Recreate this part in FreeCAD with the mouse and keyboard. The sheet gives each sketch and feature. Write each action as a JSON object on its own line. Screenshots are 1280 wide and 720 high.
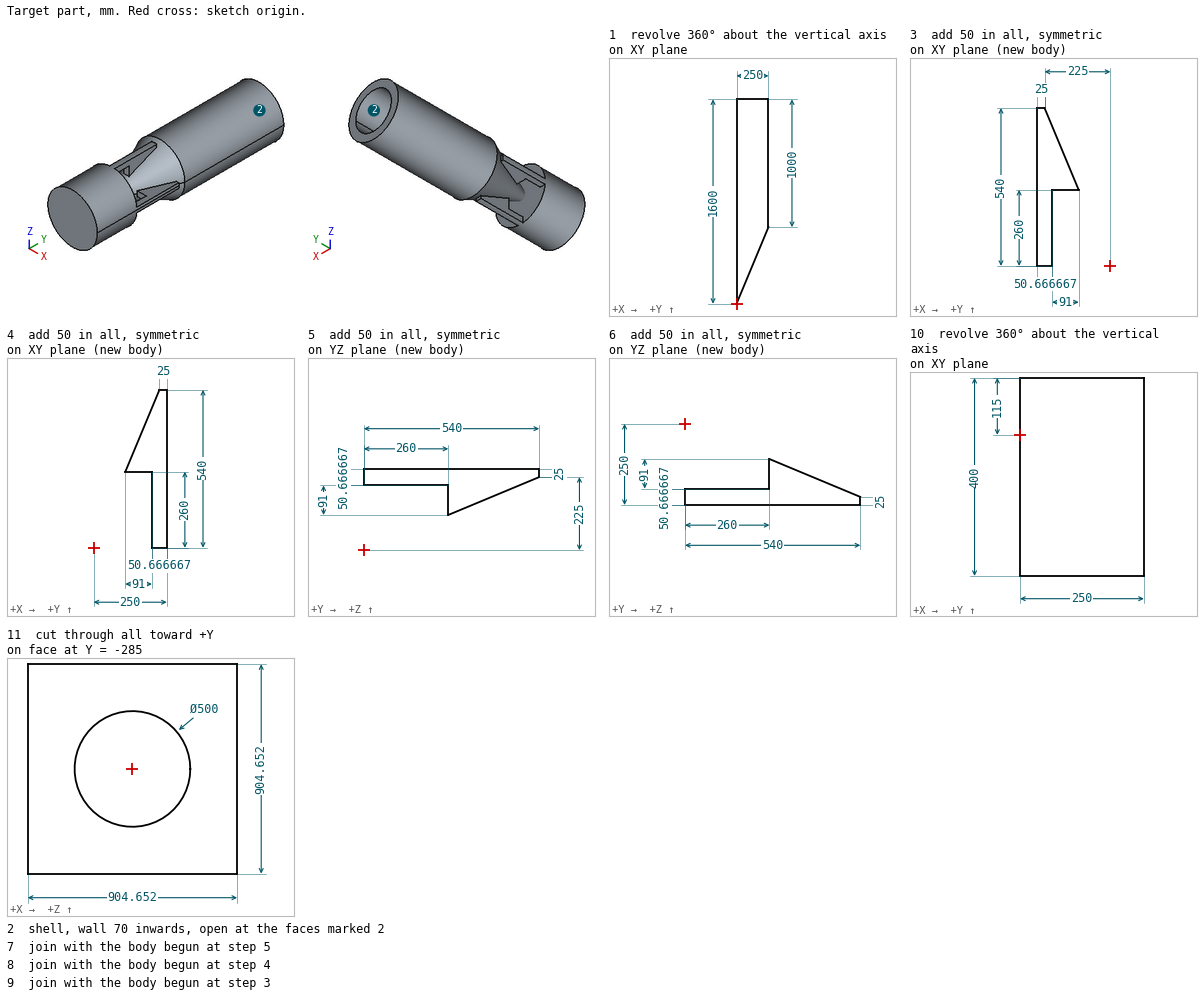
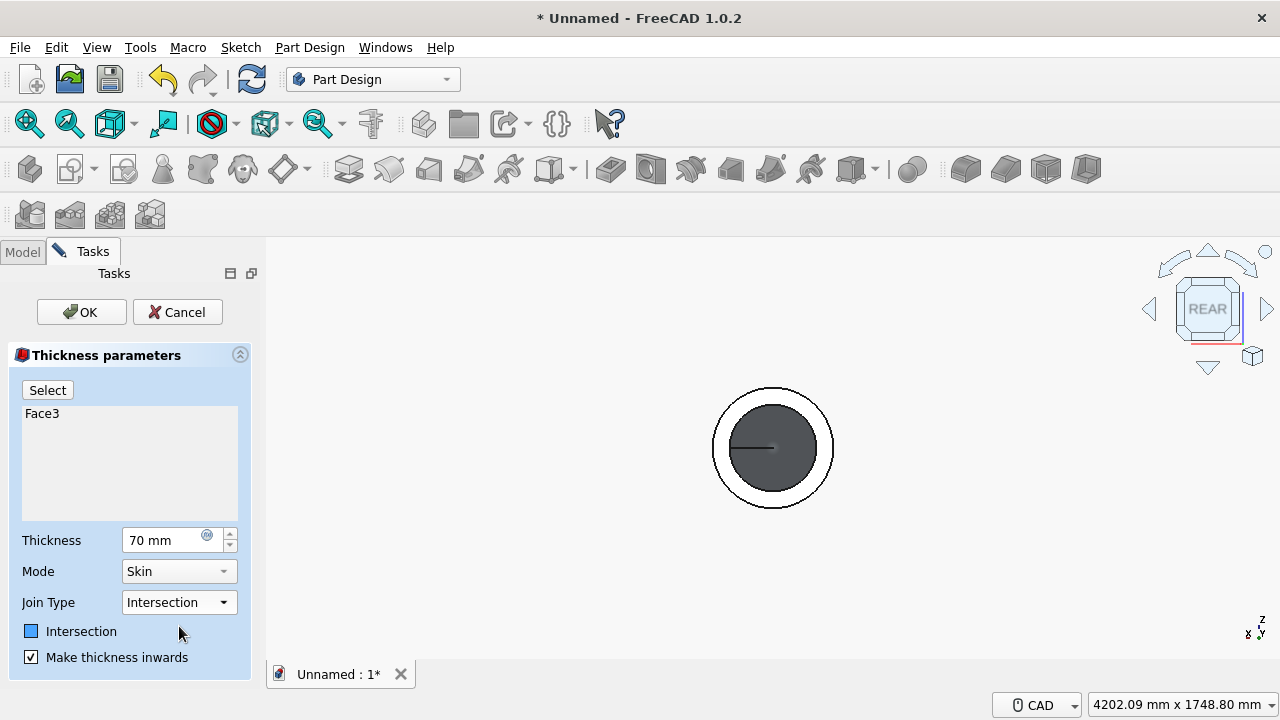
{"action": "left_click", "coordinate": [82, 312]}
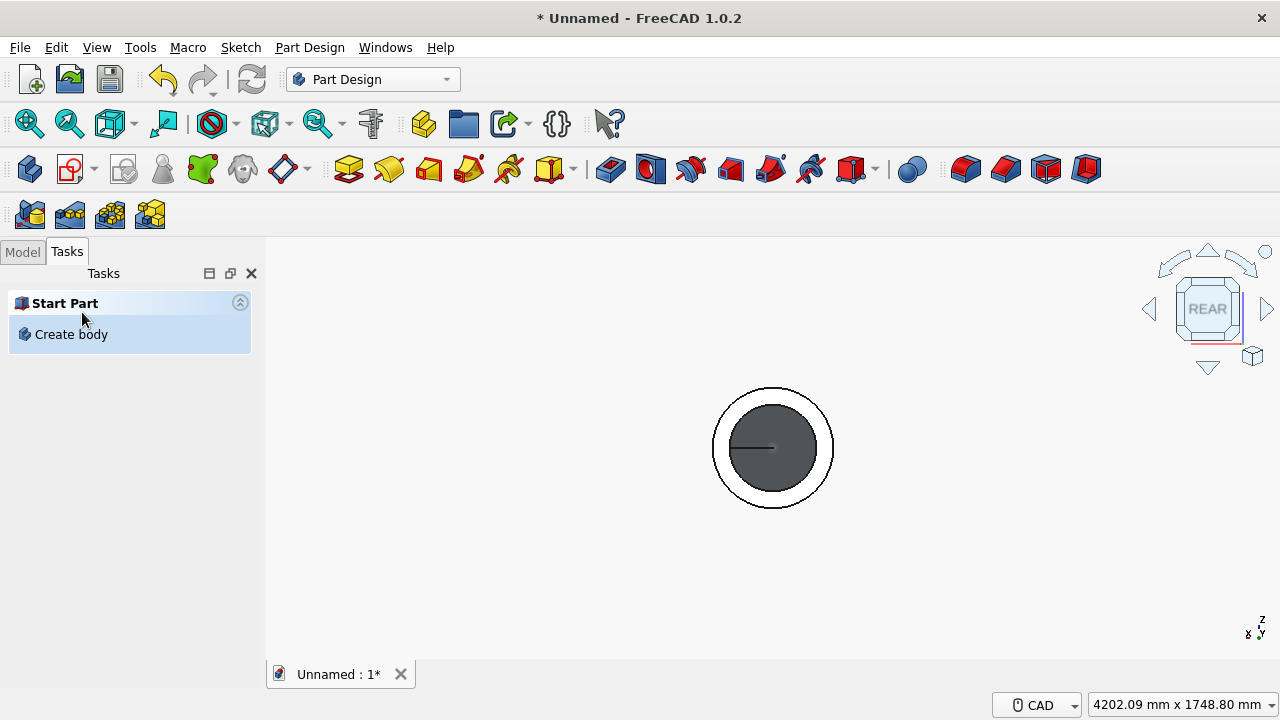
{"action": "left_click", "coordinate": [30, 124]}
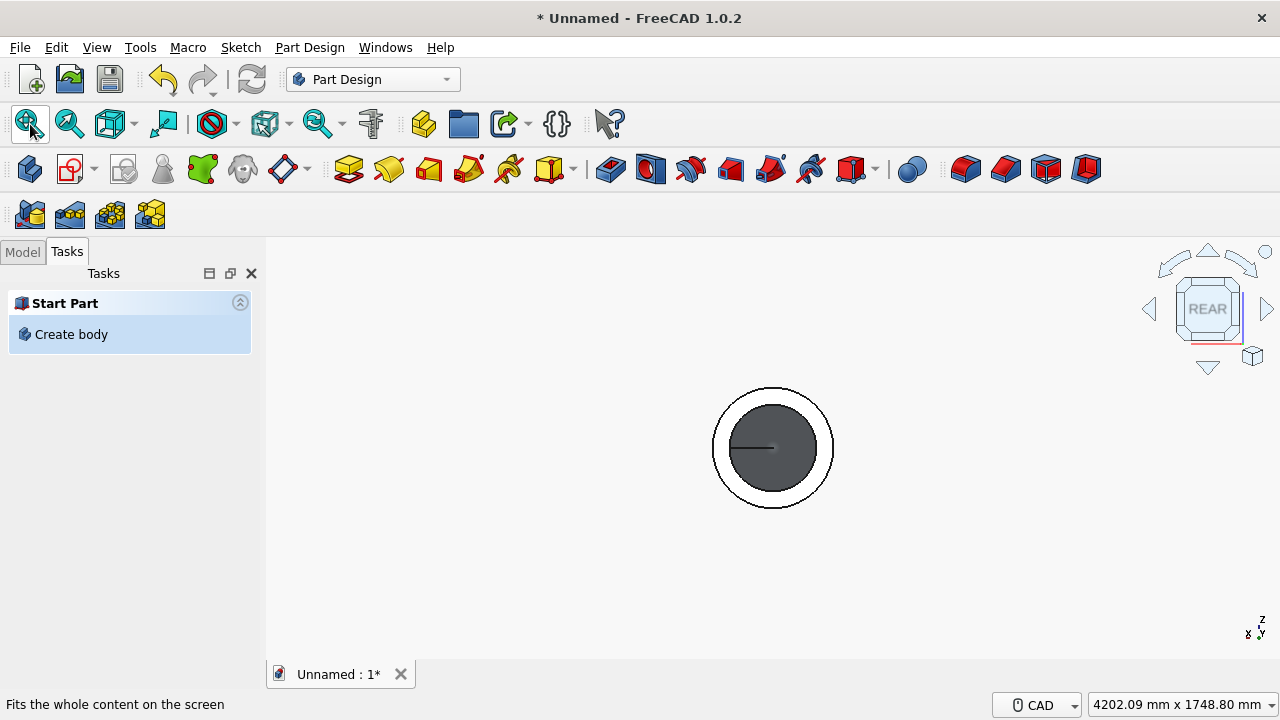
{"action": "left_click", "coordinate": [30, 170]}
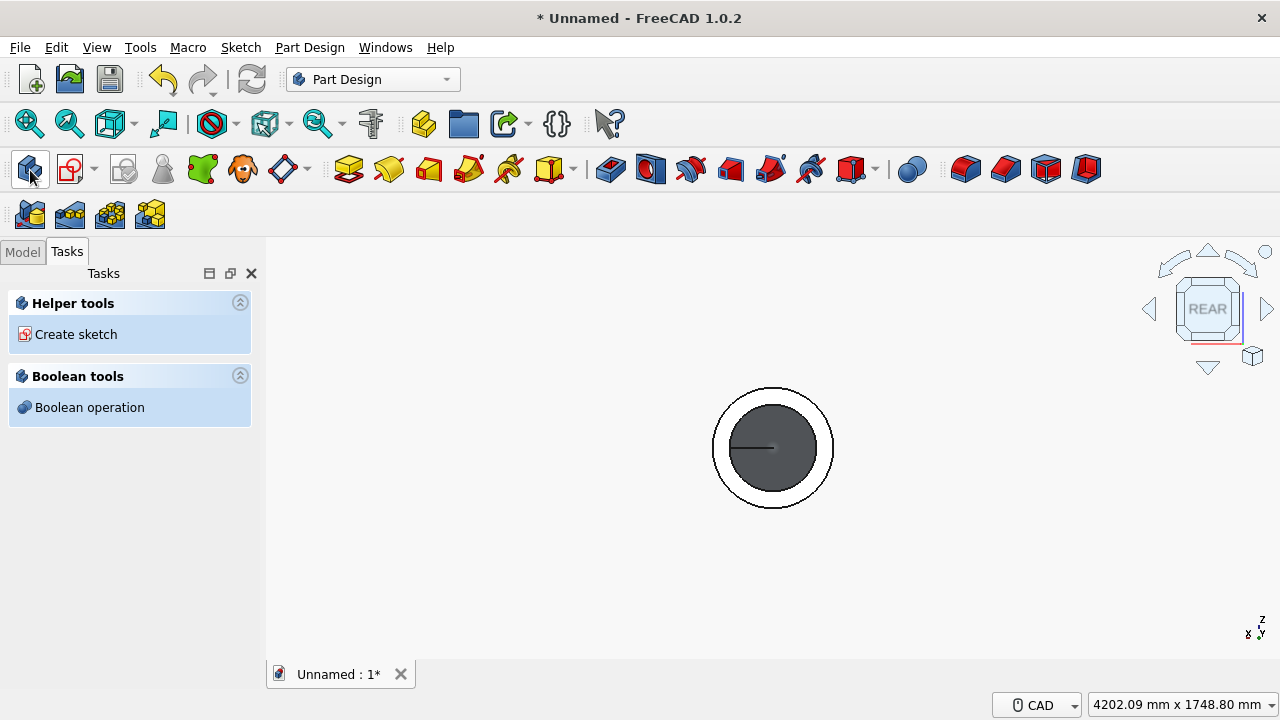
{"action": "left_click", "coordinate": [306, 619]}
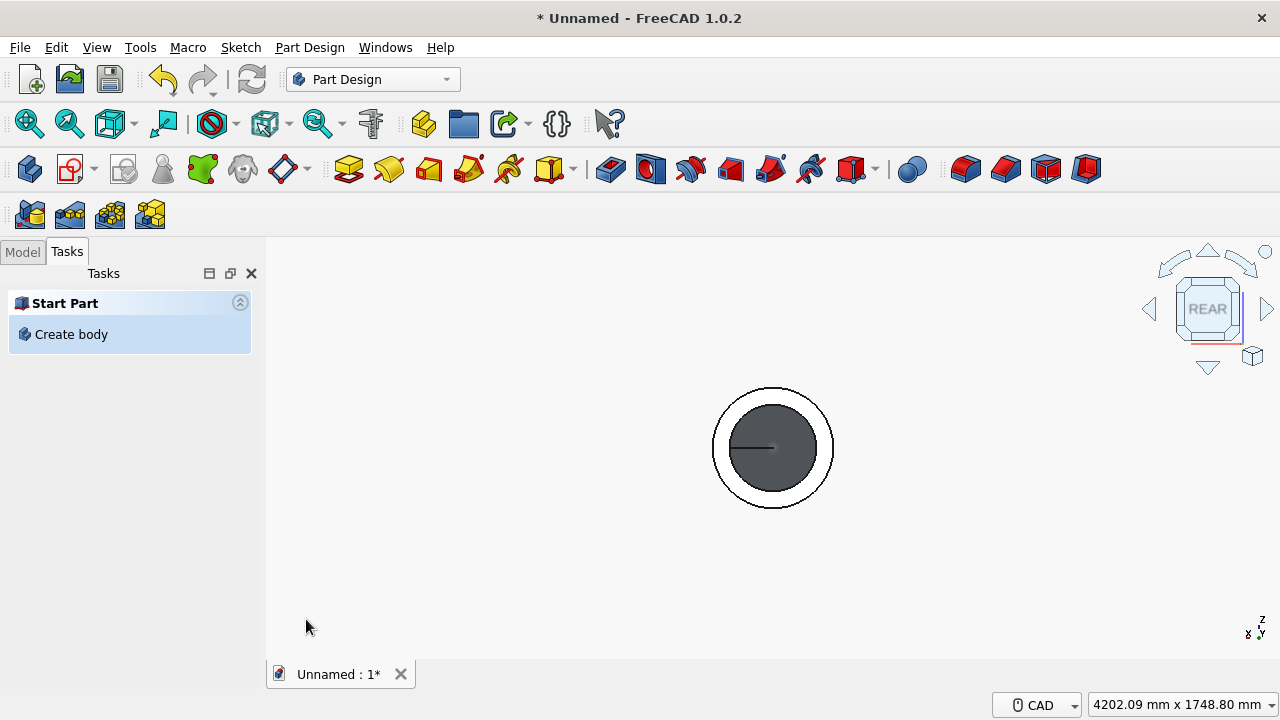
{"action": "left_click", "coordinate": [70, 170]}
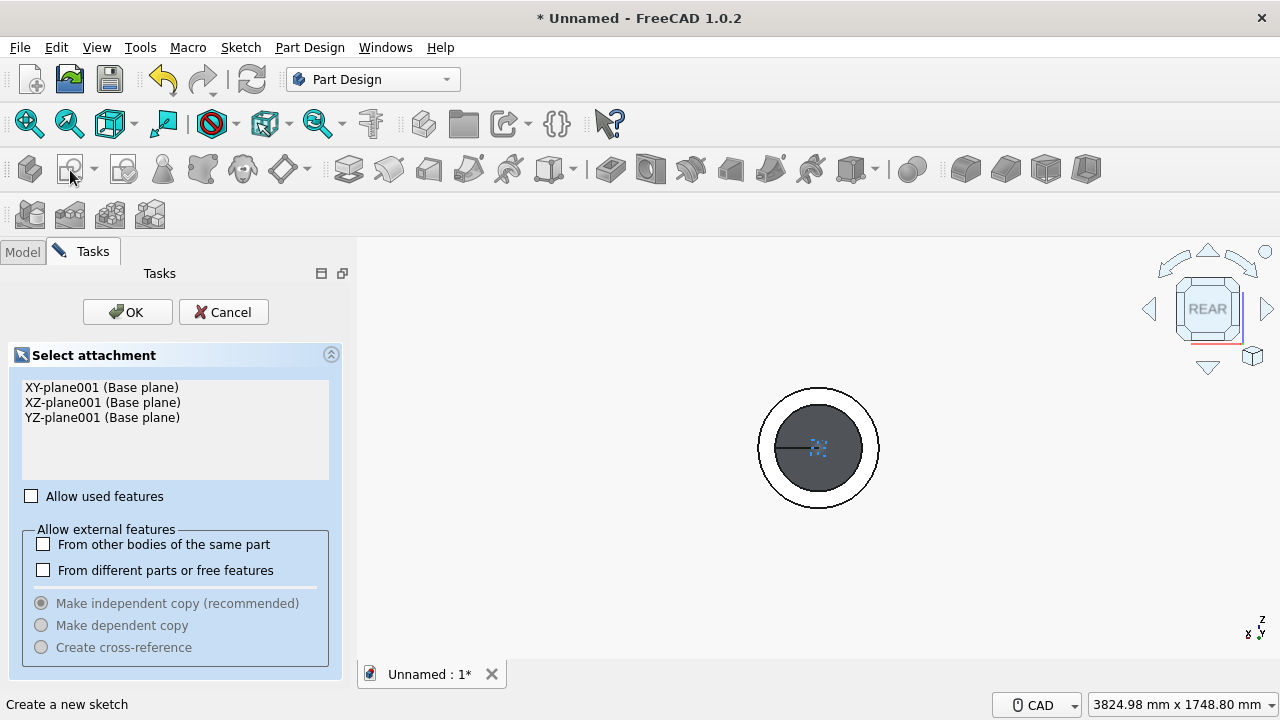
{"action": "left_click", "coordinate": [82, 388]}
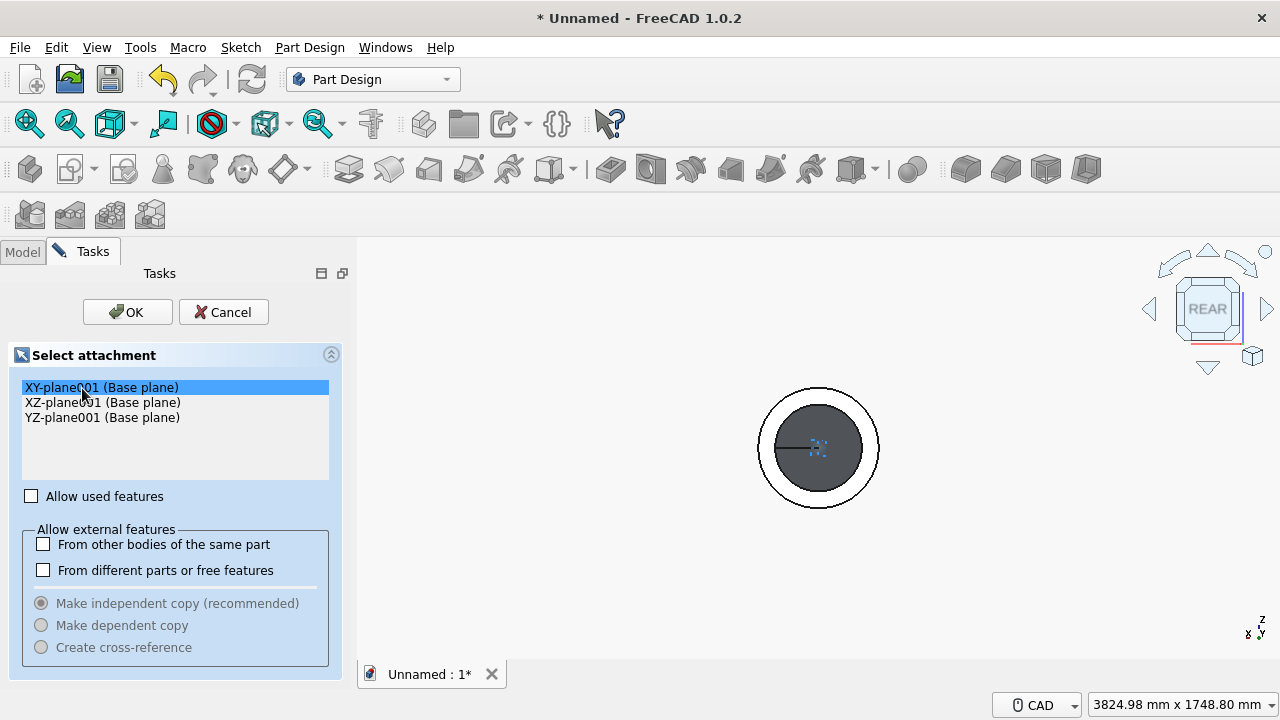
{"action": "left_click", "coordinate": [128, 312]}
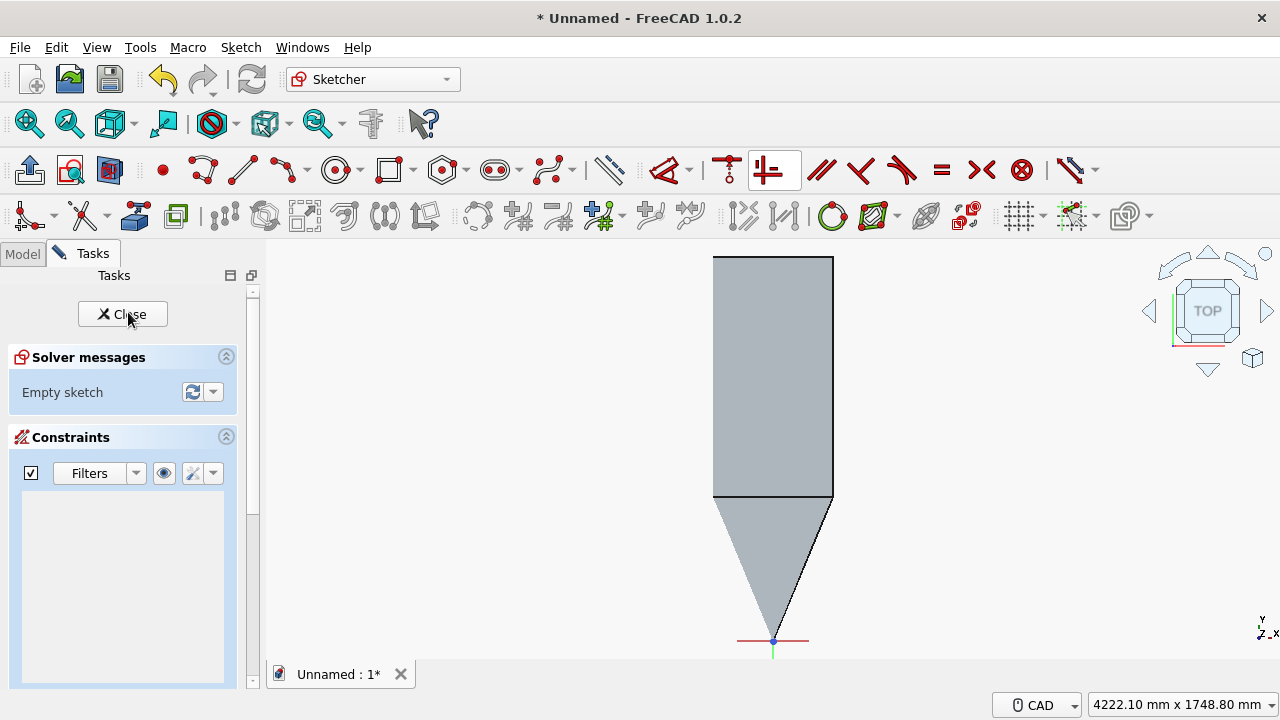
{"action": "scroll", "coordinate": [704, 449], "scroll_direction": "down", "scroll_amount": 5}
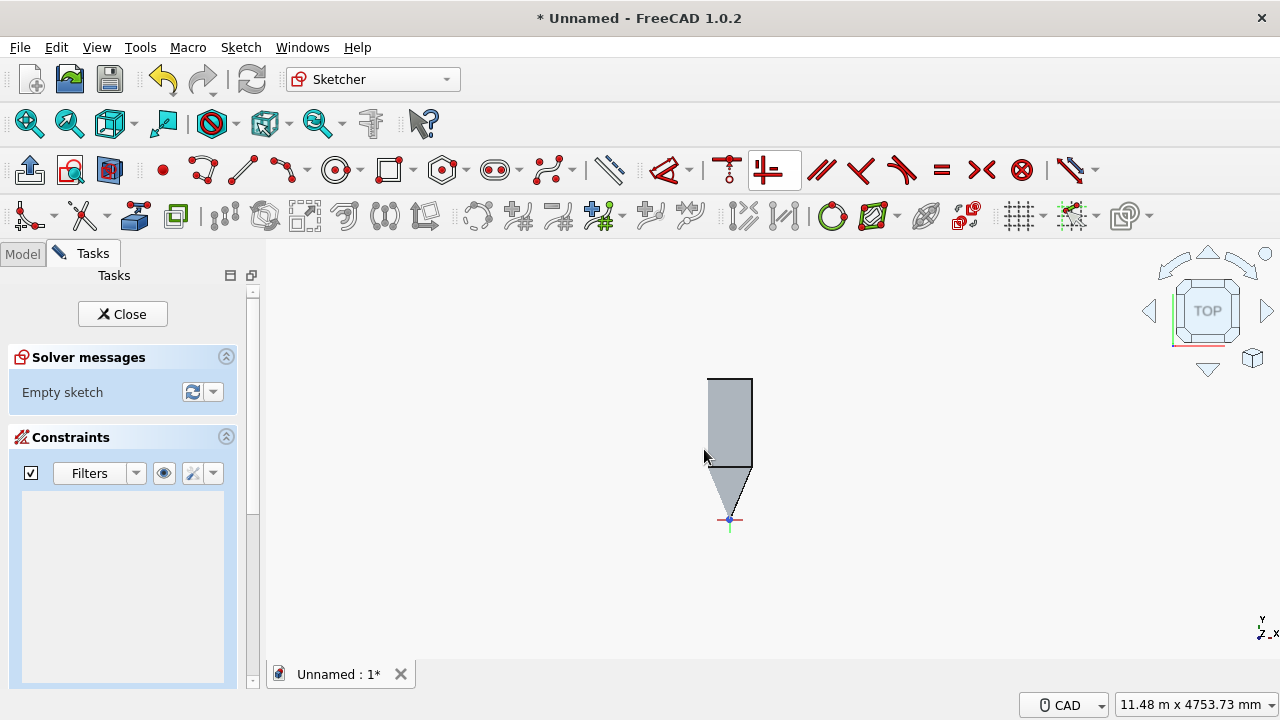
{"action": "scroll", "coordinate": [722, 508], "scroll_direction": "up", "scroll_amount": 8}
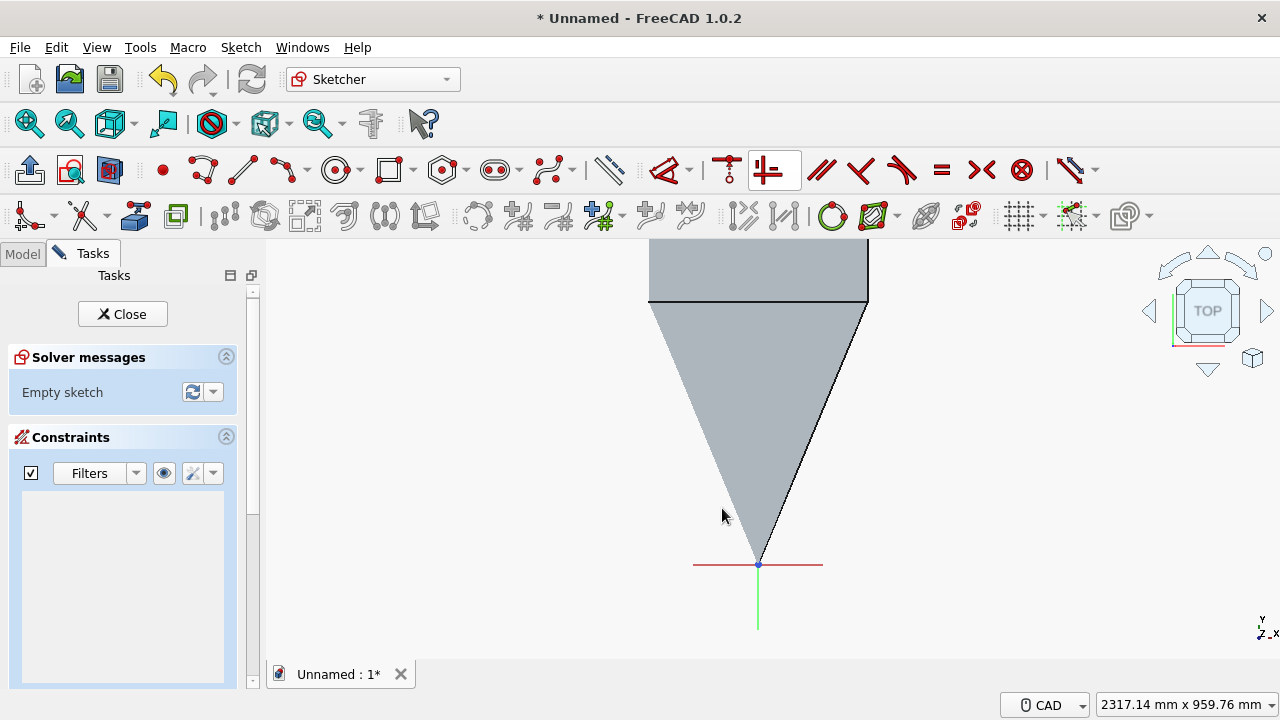
{"action": "left_click", "coordinate": [204, 170]}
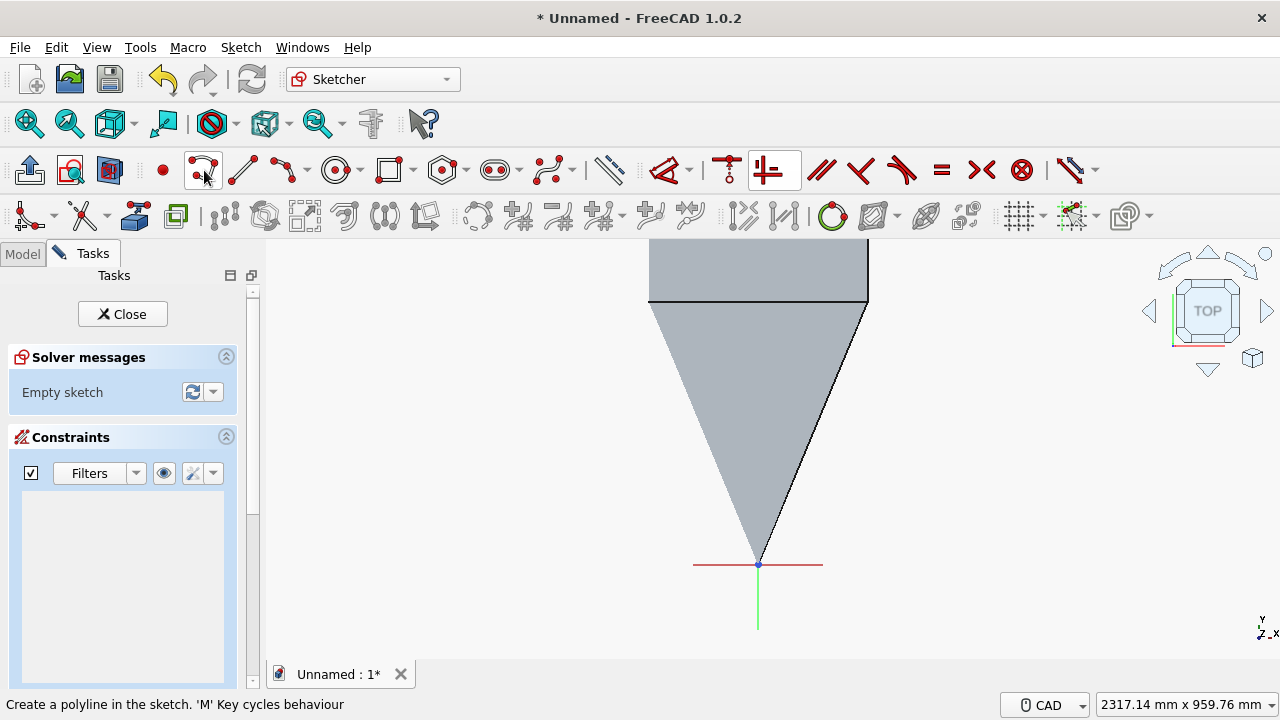
{"action": "left_click", "coordinate": [671, 565]}
{"action": "left_click", "coordinate": [671, 451]}
{"action": "left_click", "coordinate": [711, 451]}
{"action": "left_click", "coordinate": [660, 329]}